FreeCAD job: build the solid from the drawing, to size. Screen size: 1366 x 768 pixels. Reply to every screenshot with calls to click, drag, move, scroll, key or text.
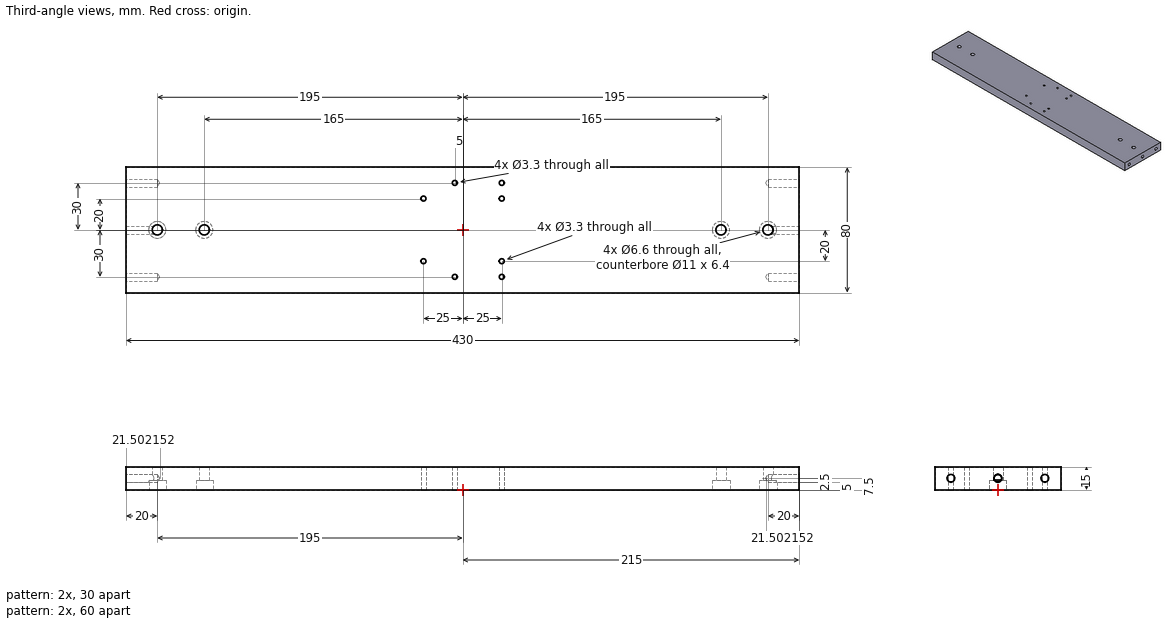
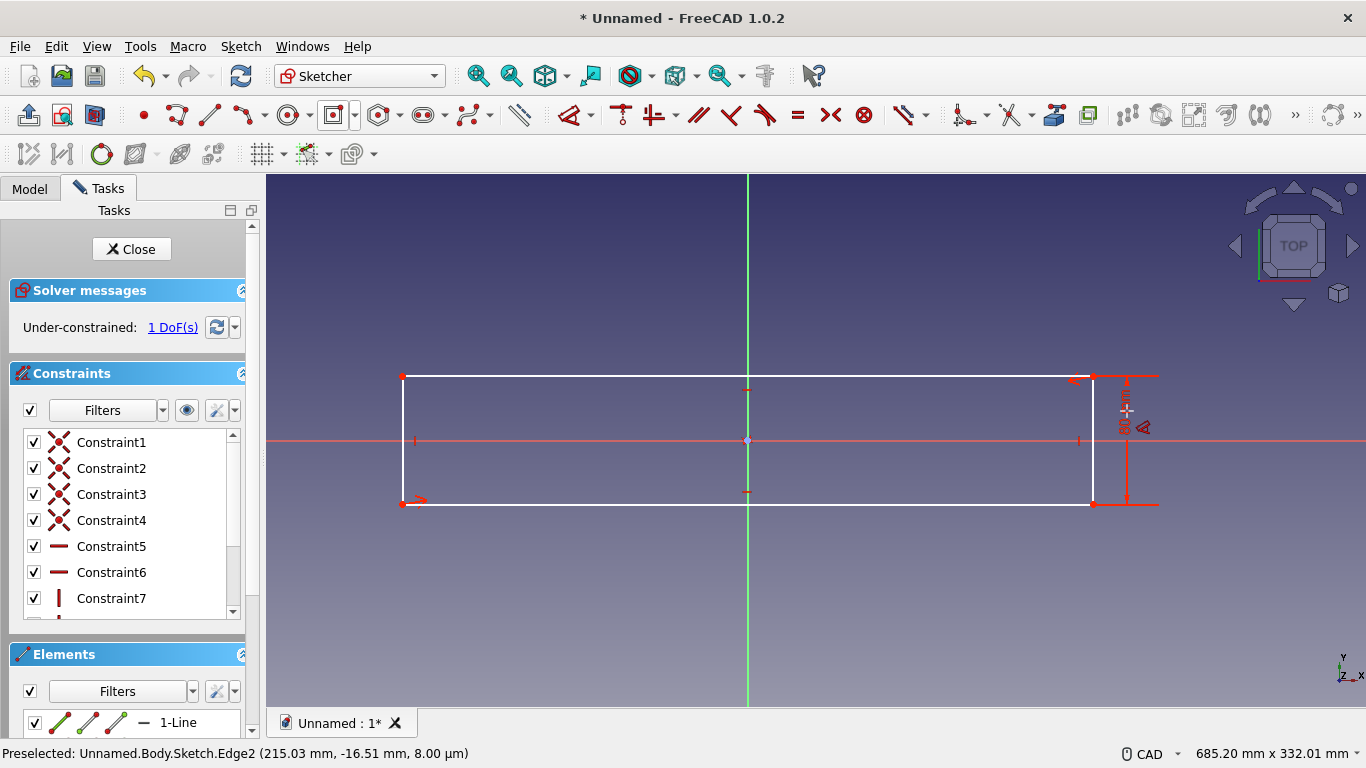
click(610, 505)
click(589, 539)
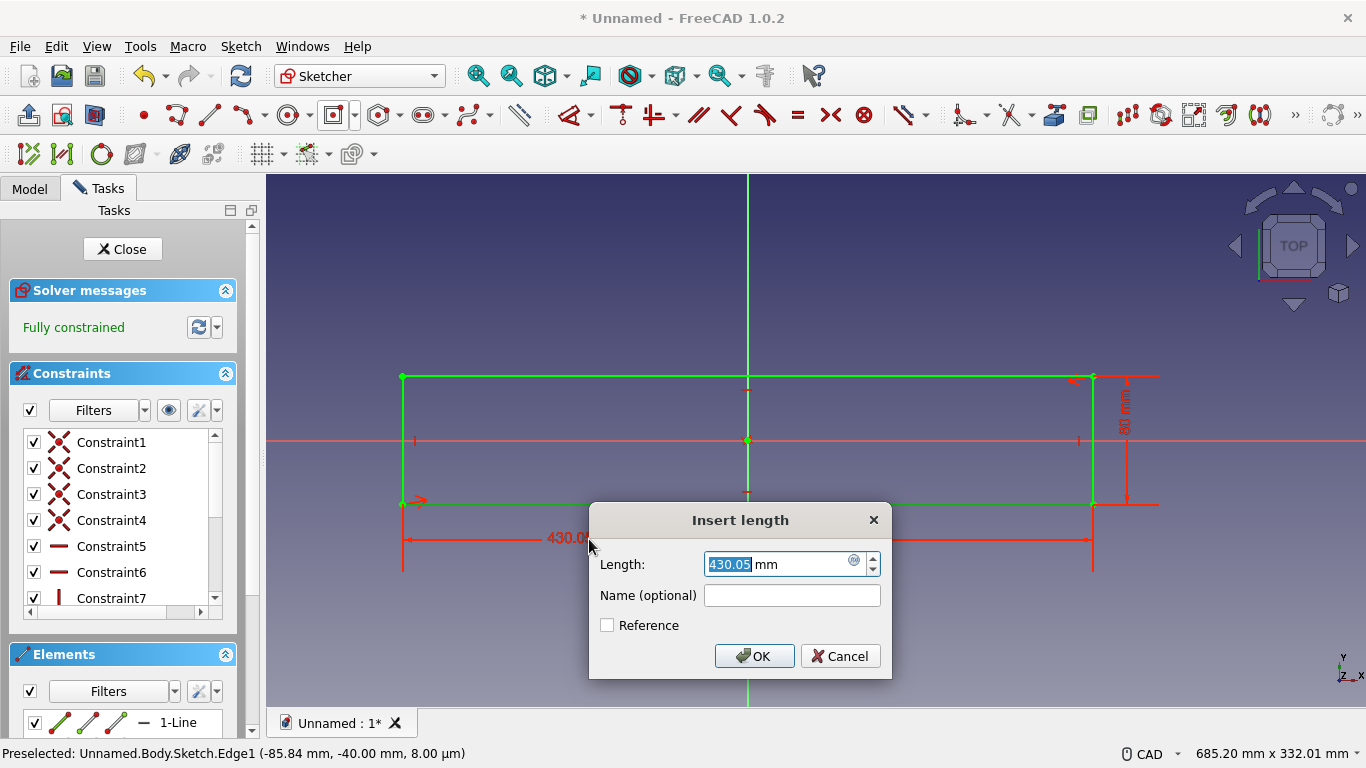
text(430)
key(Return)
key(Escape)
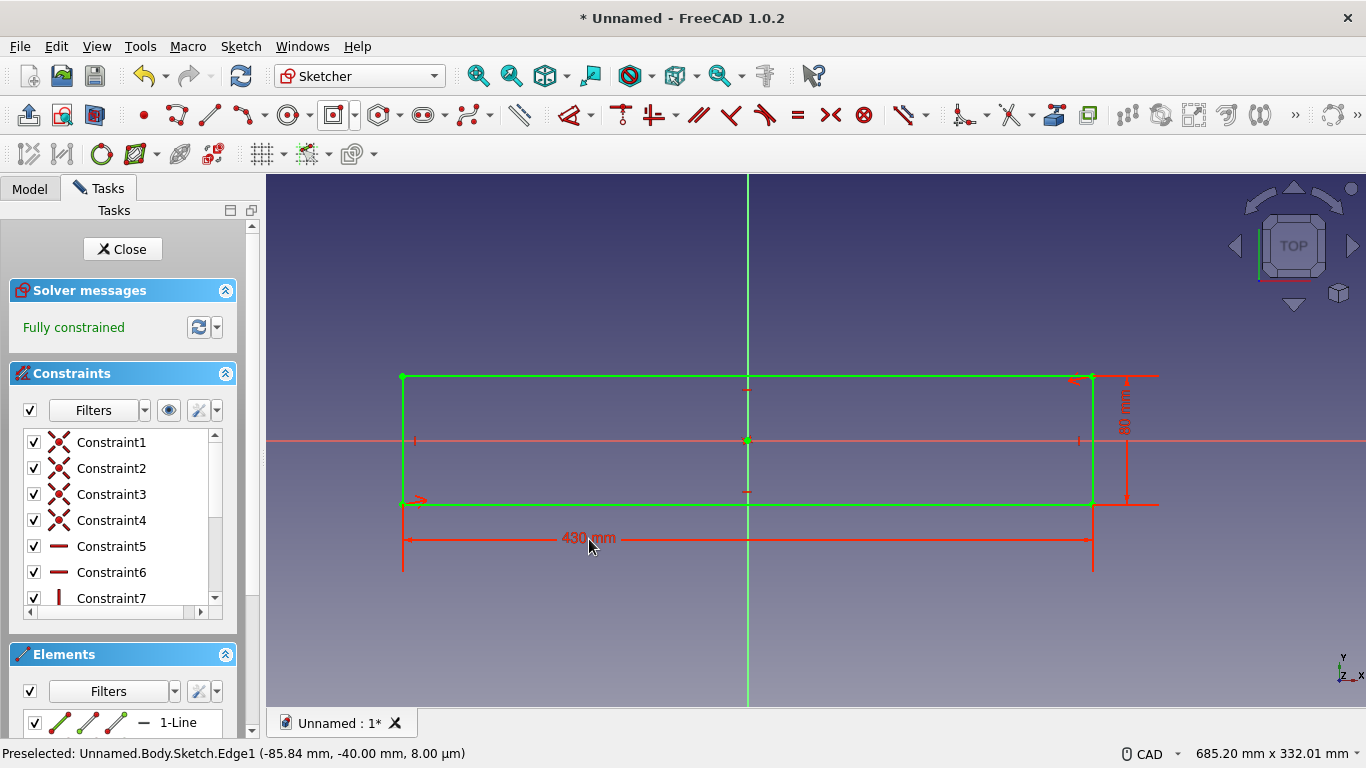
click(123, 249)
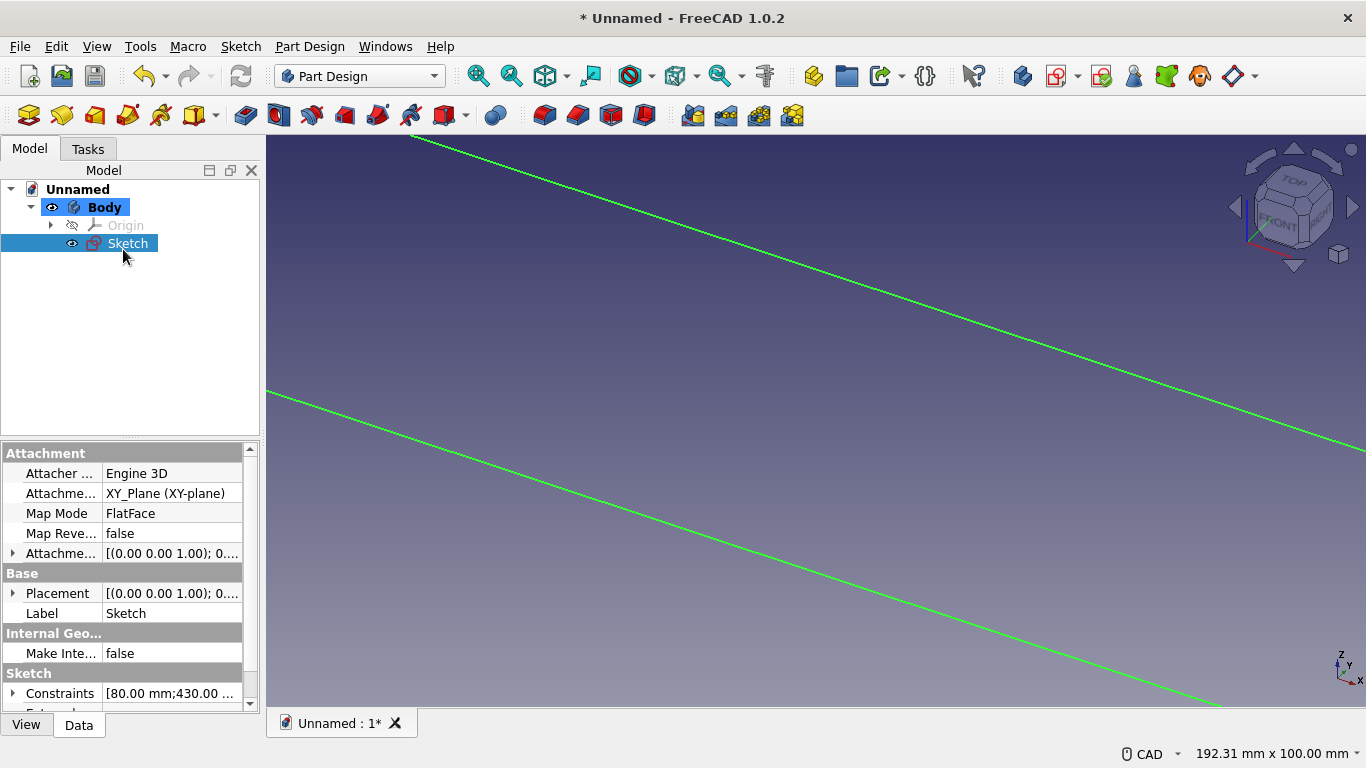
click(29, 116)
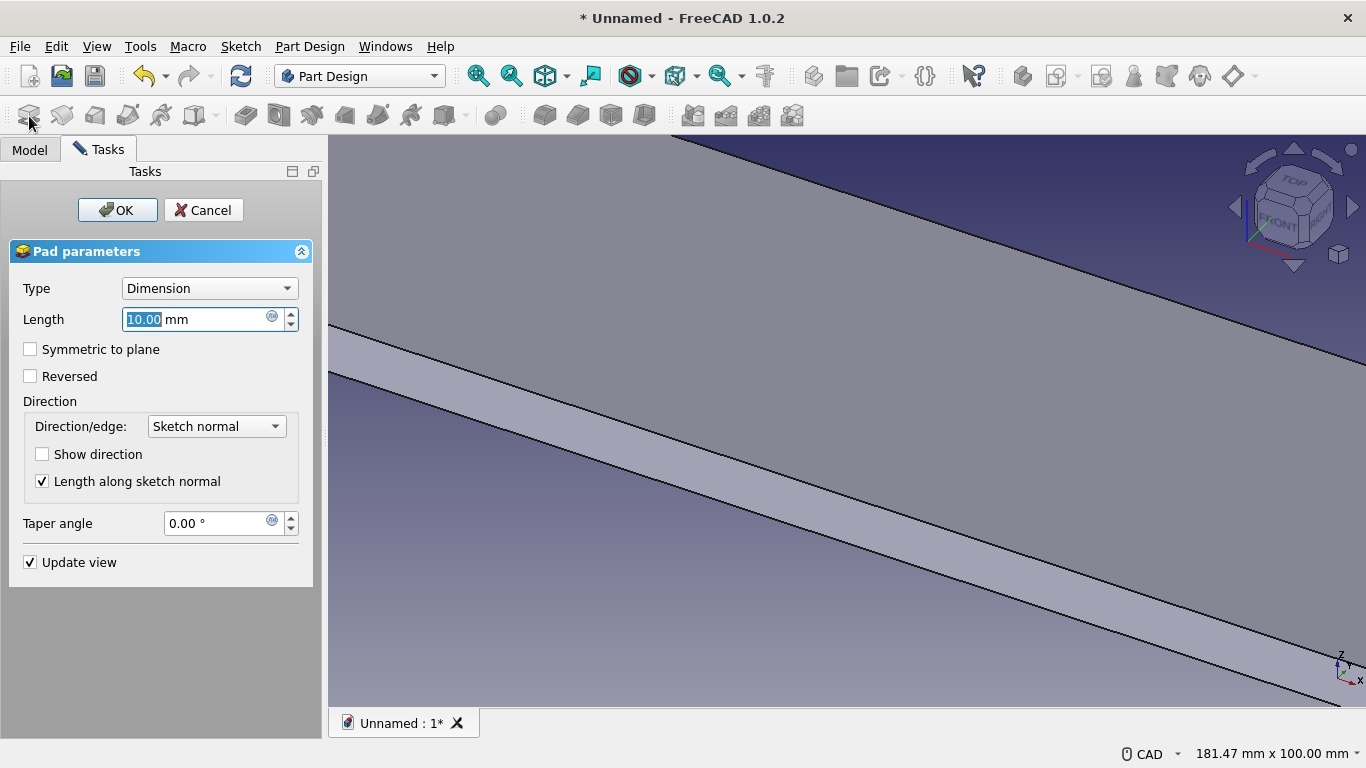
text(15)
key(Tab)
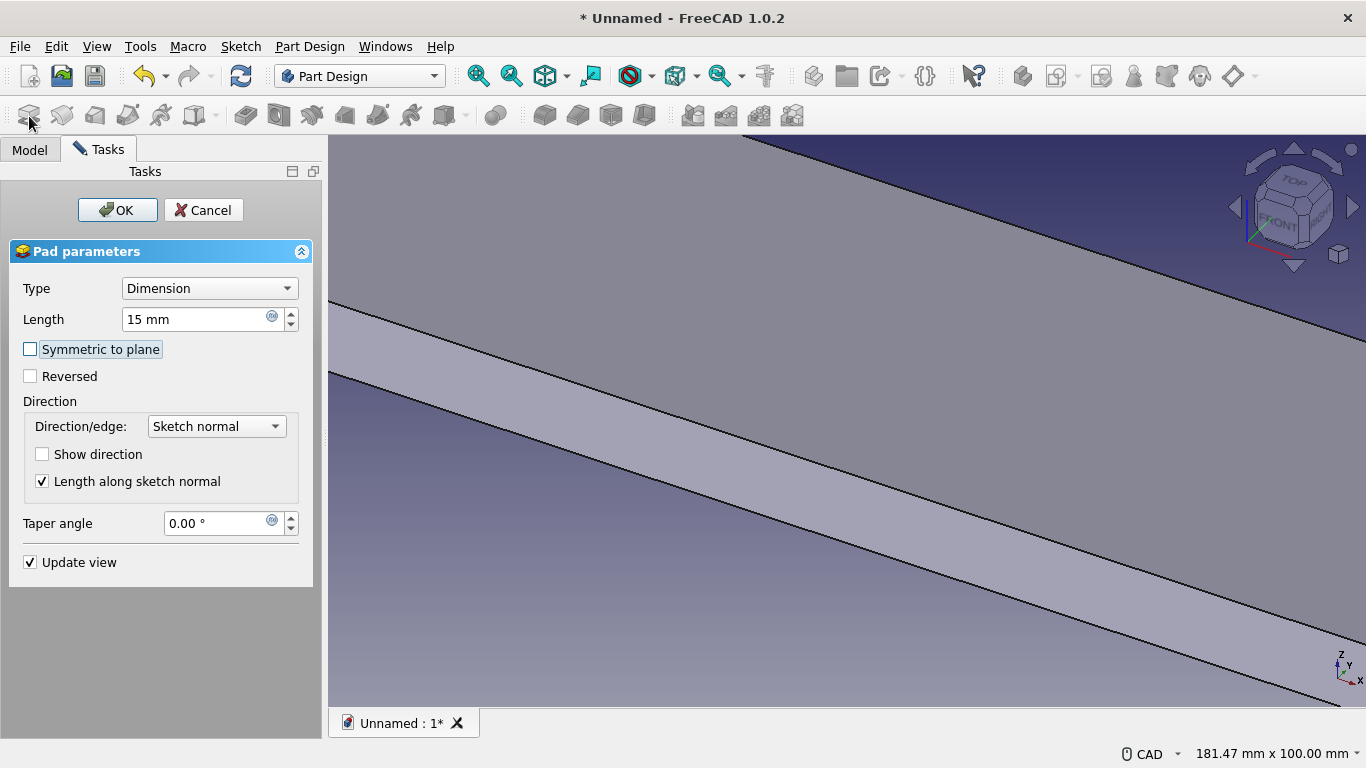
click(118, 210)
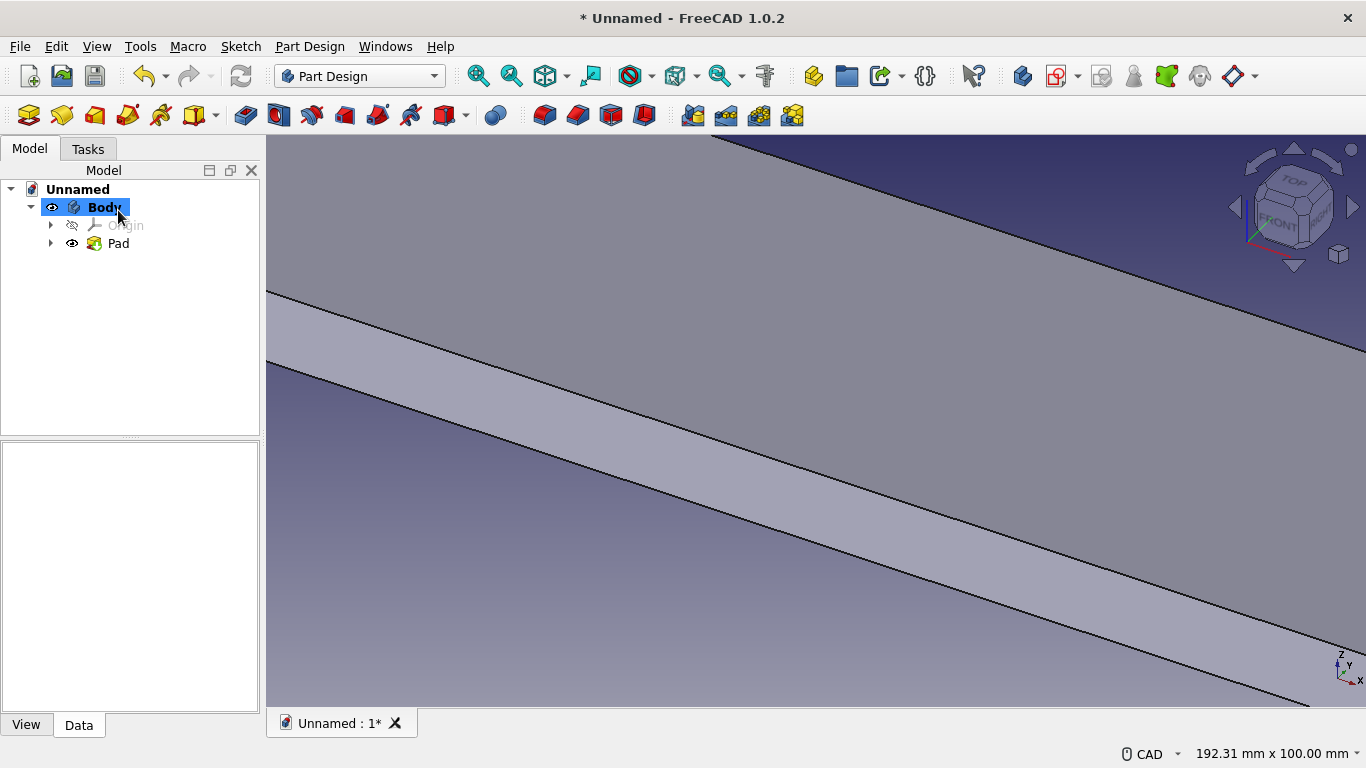
key(v)
key(f)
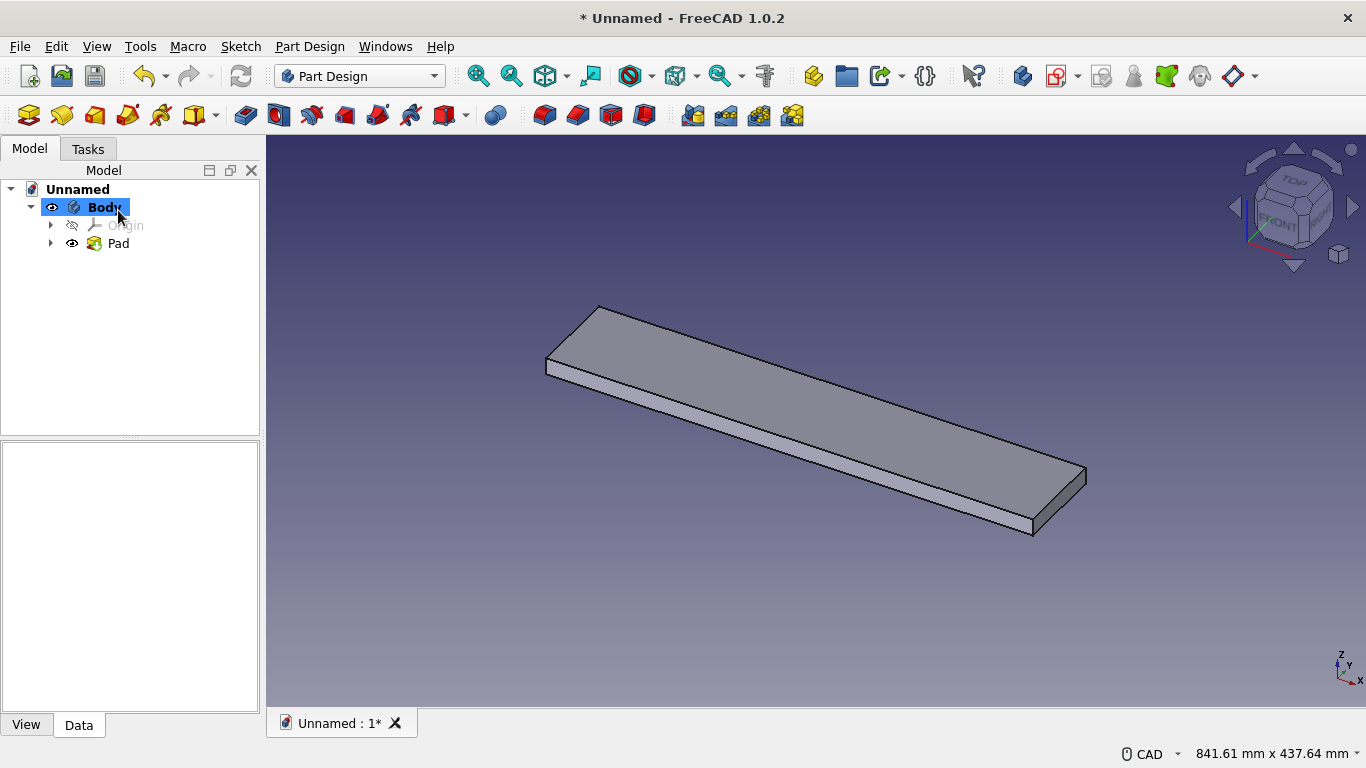
click(1056, 76)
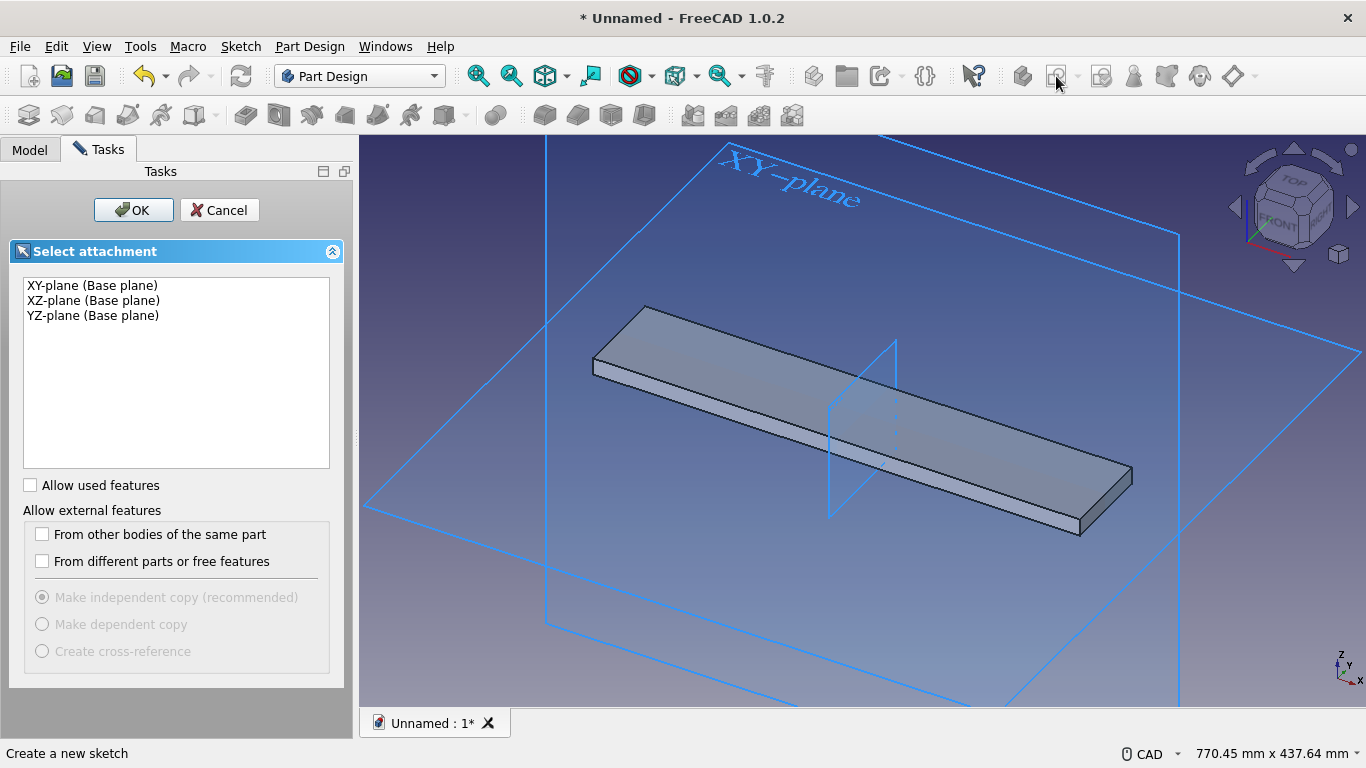
click(84, 286)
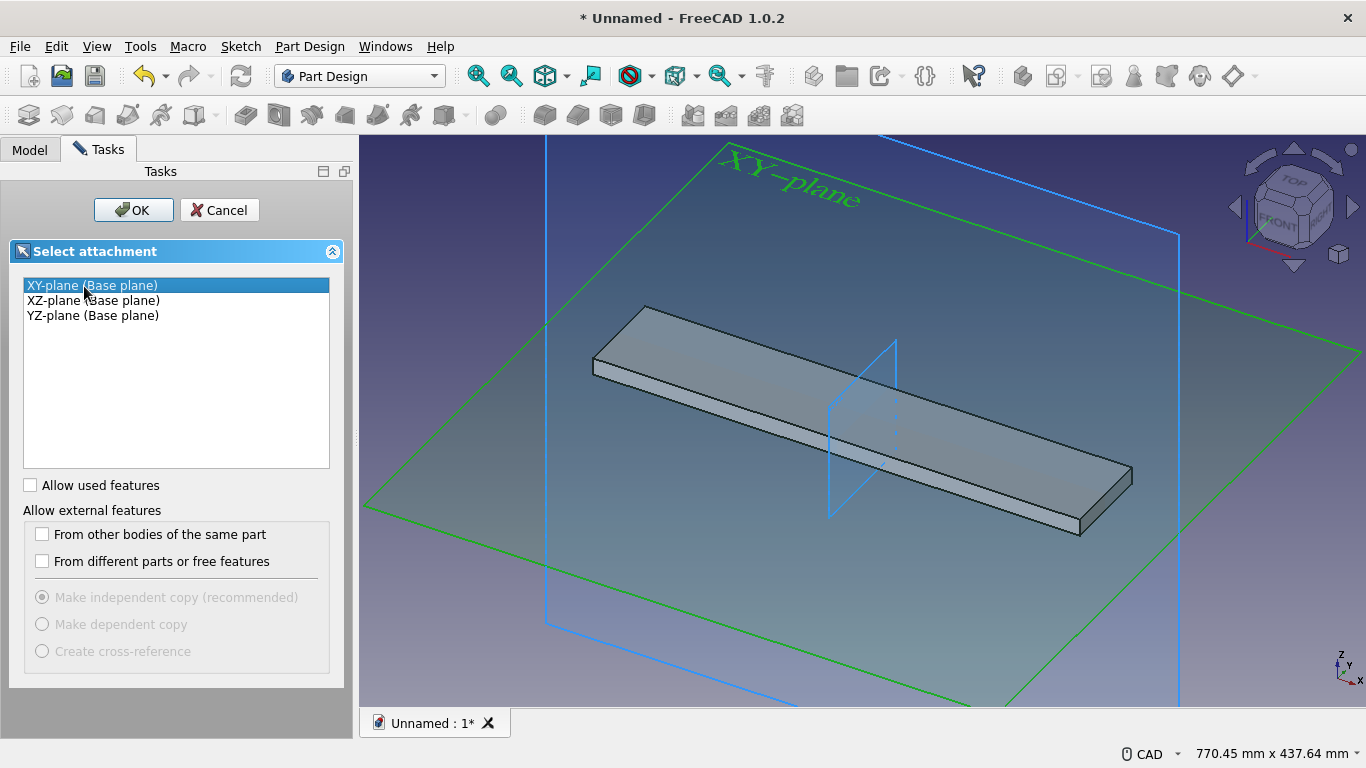
click(134, 210)